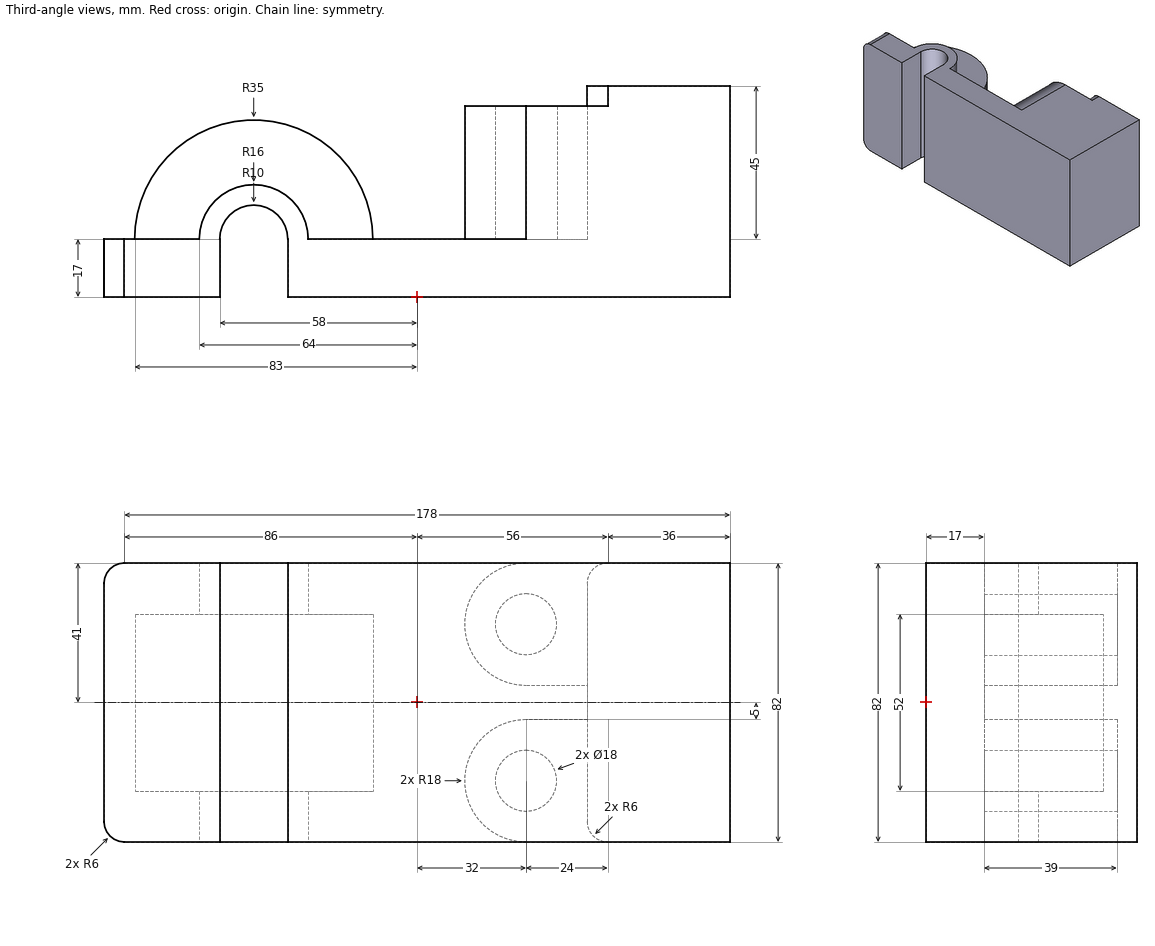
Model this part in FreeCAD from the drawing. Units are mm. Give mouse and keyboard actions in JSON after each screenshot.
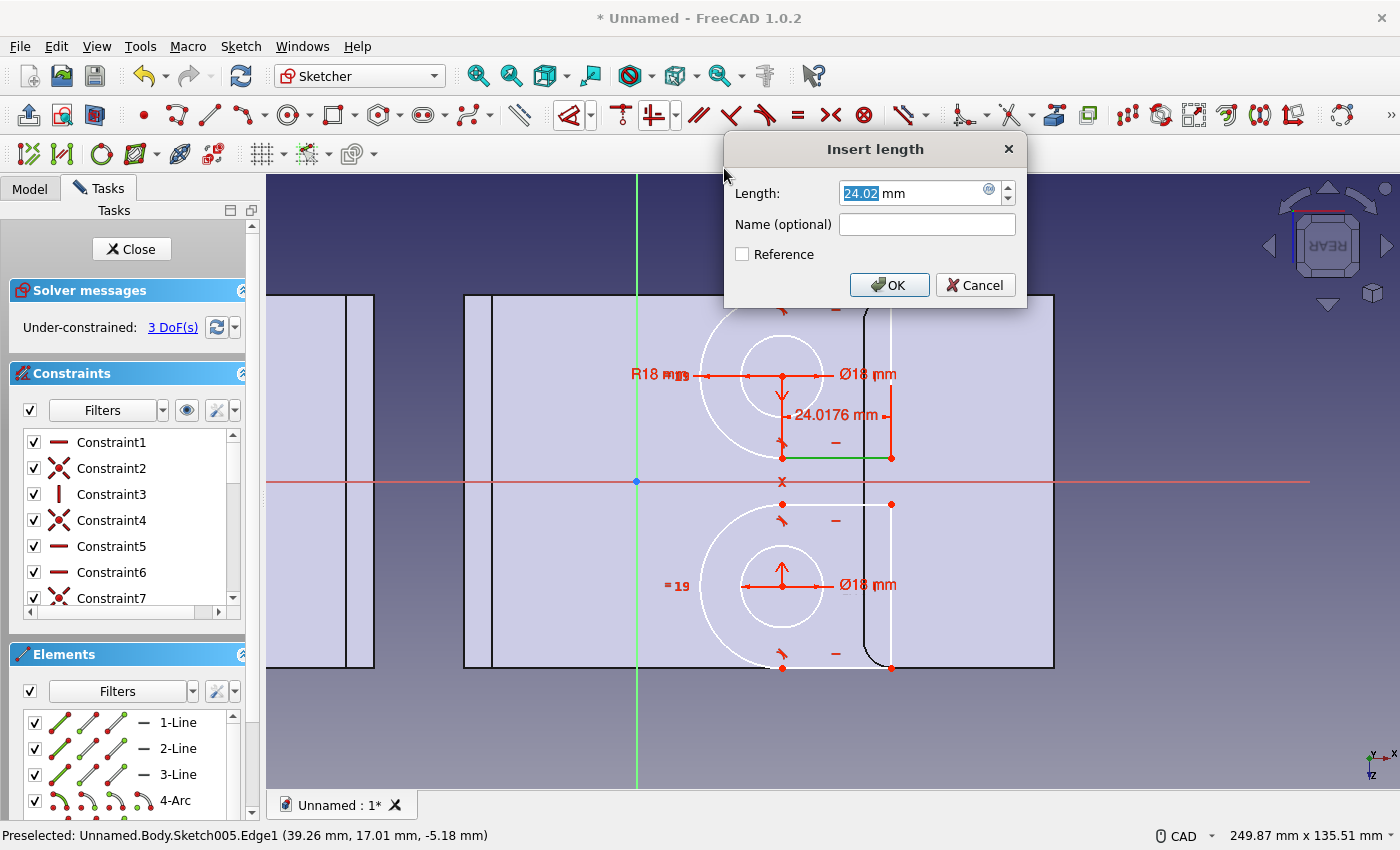
{"action": "type", "text": "24"}
{"action": "key", "text": "Return"}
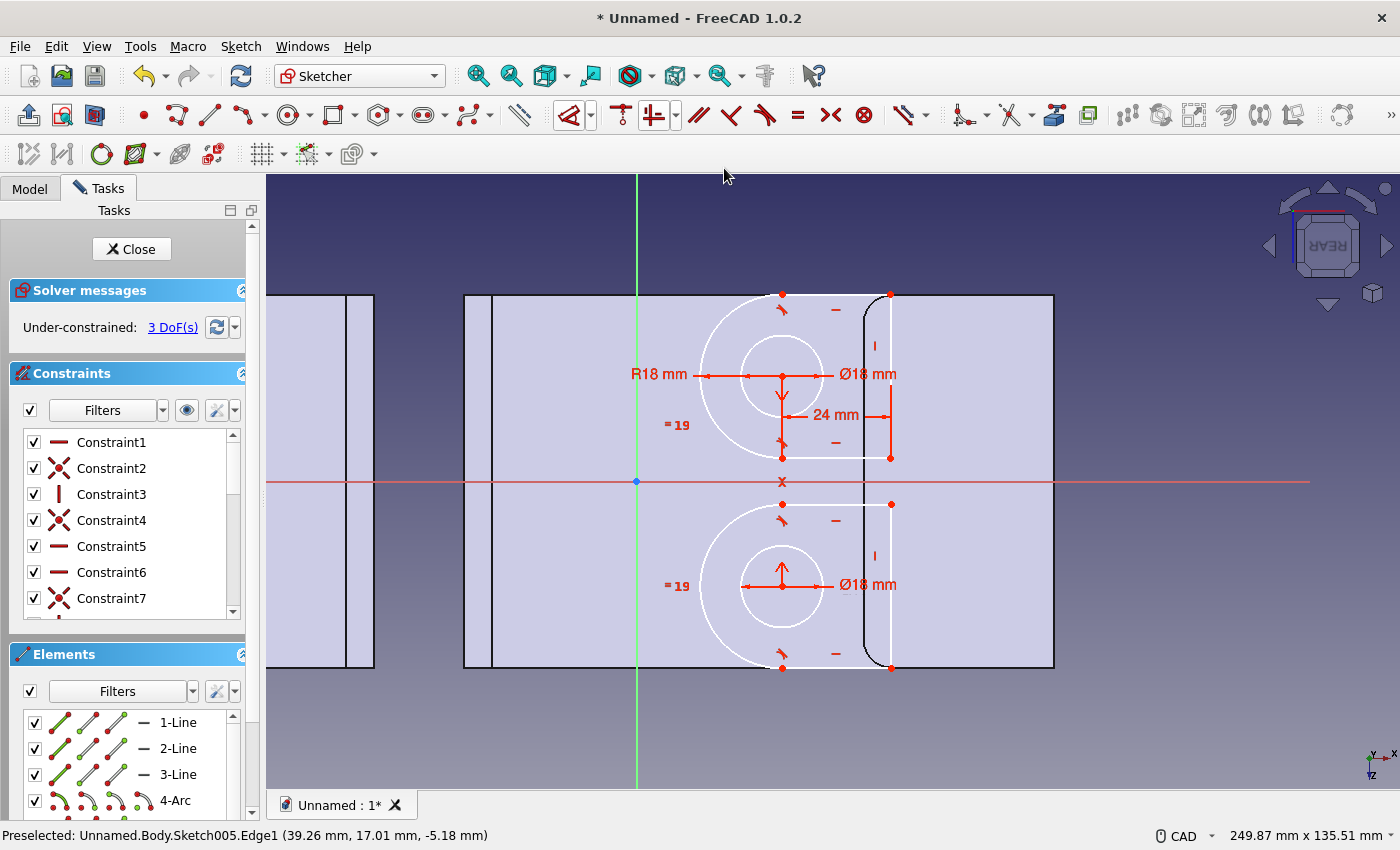
{"action": "left_click", "coordinate": [815, 668]}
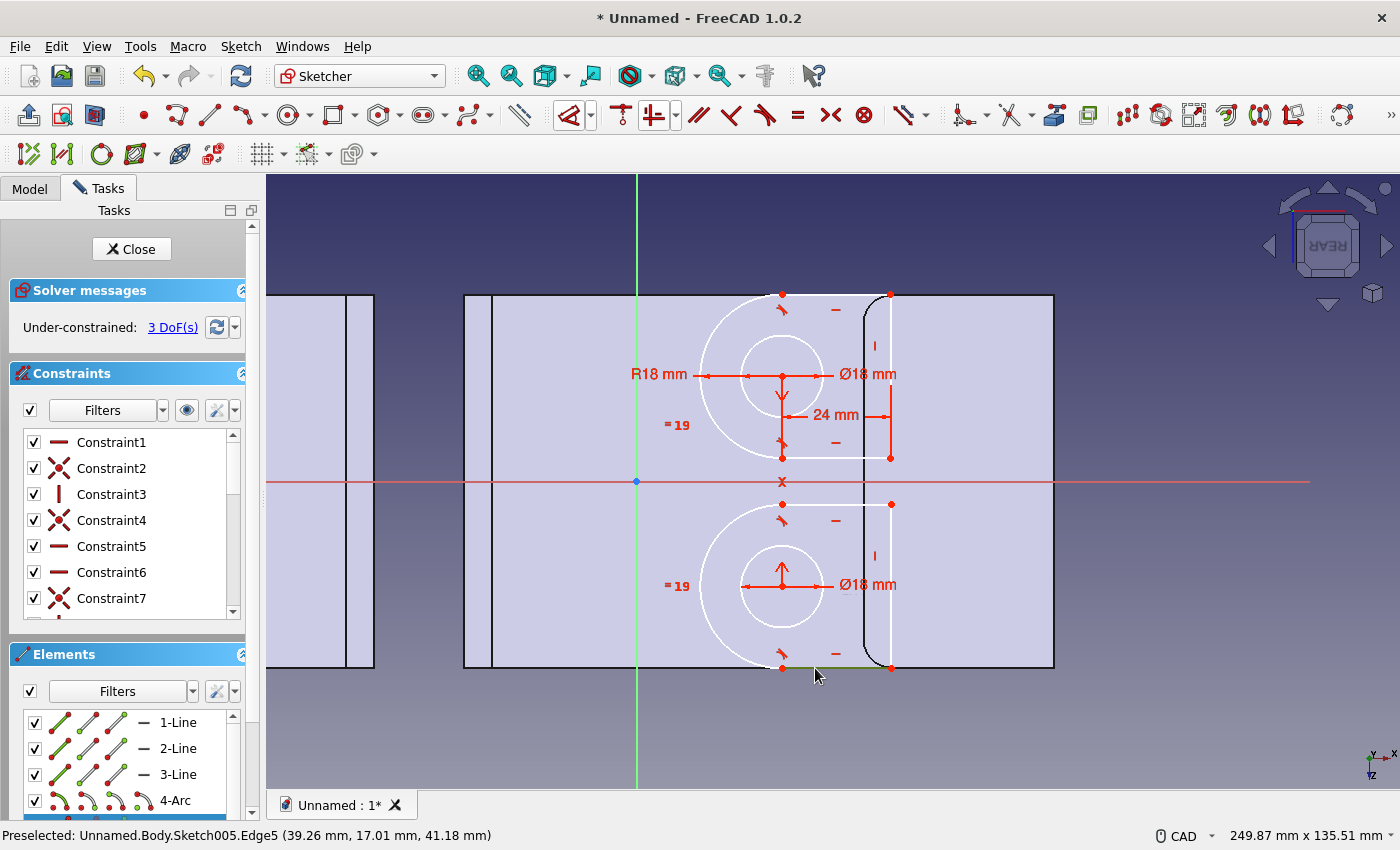
{"action": "key", "text": "l"}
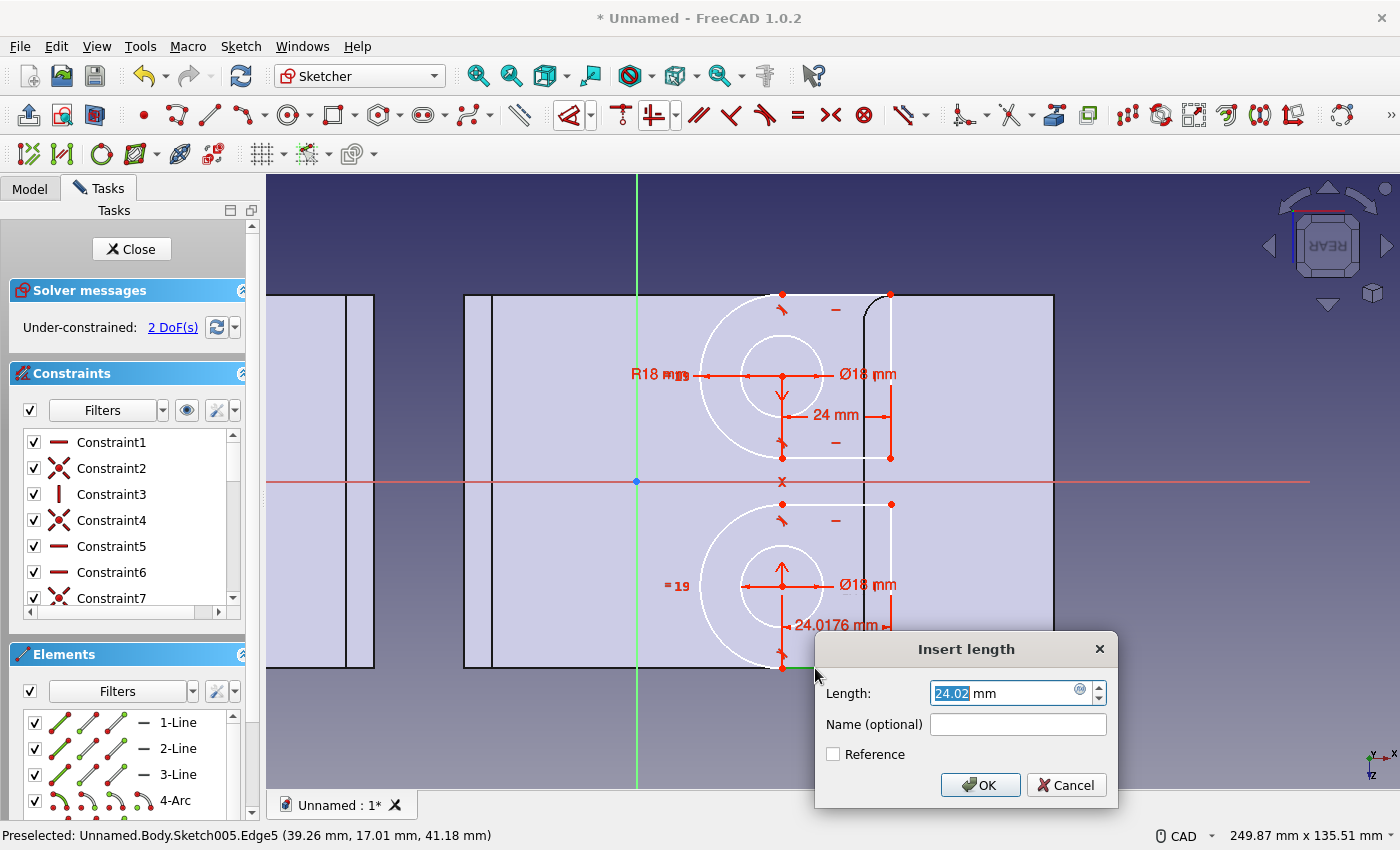
{"action": "type", "text": "24"}
{"action": "key", "text": "Return"}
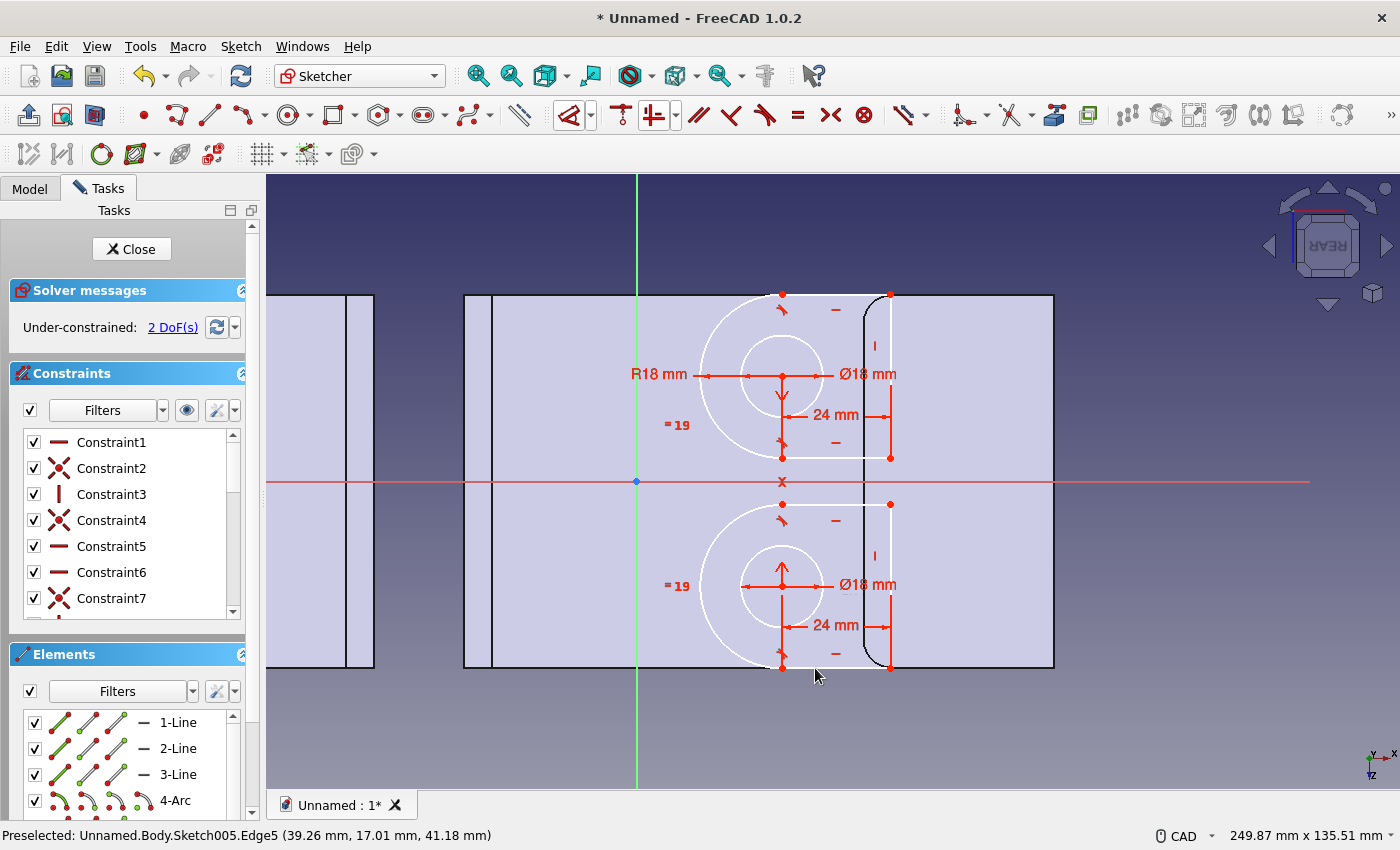
{"action": "scroll", "coordinate": [782, 458], "scroll_direction": "up", "scroll_amount": 3}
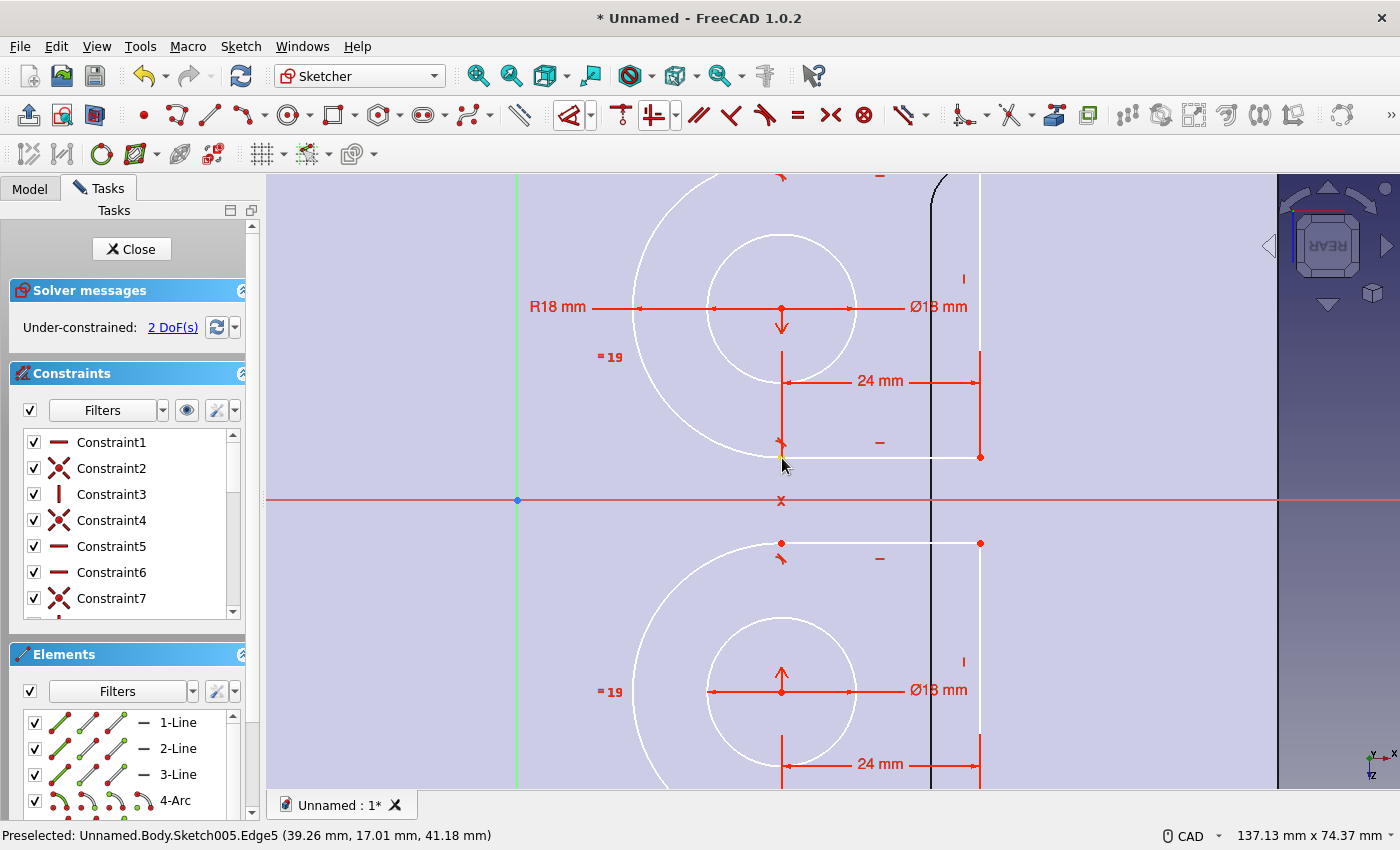
{"action": "left_click", "coordinate": [782, 458]}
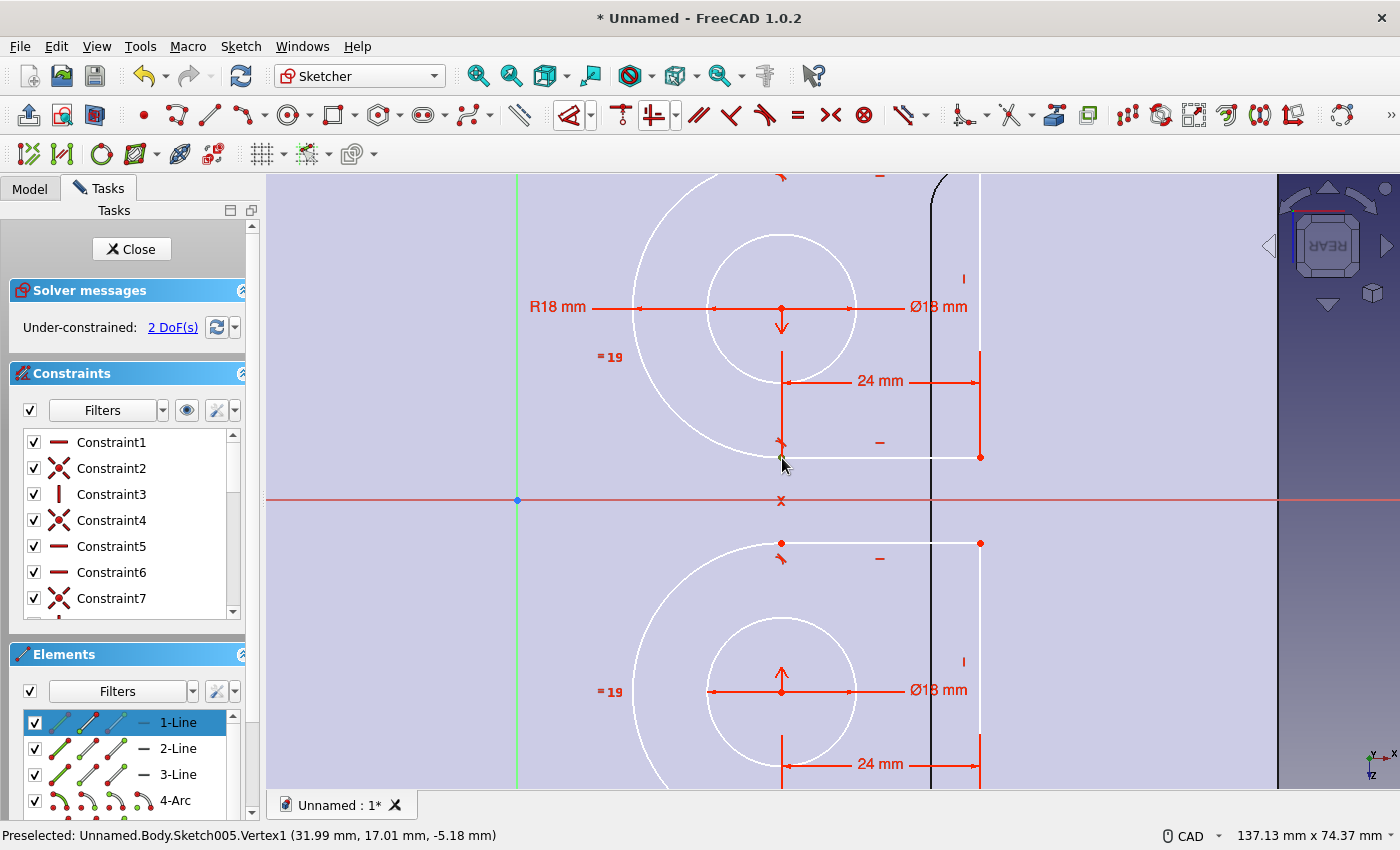
{"action": "left_click", "coordinate": [590, 116]}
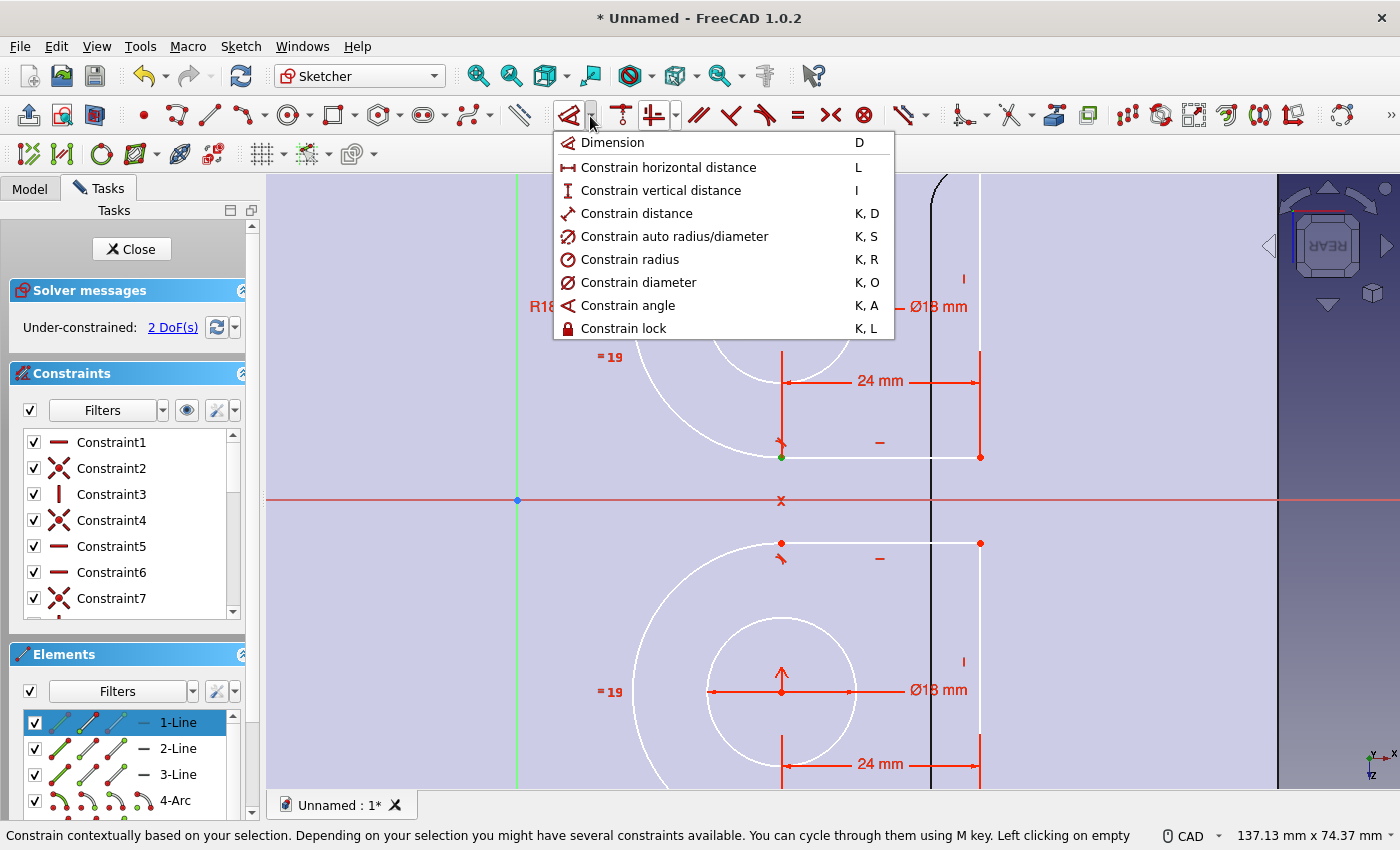
{"action": "left_click", "coordinate": [724, 190]}